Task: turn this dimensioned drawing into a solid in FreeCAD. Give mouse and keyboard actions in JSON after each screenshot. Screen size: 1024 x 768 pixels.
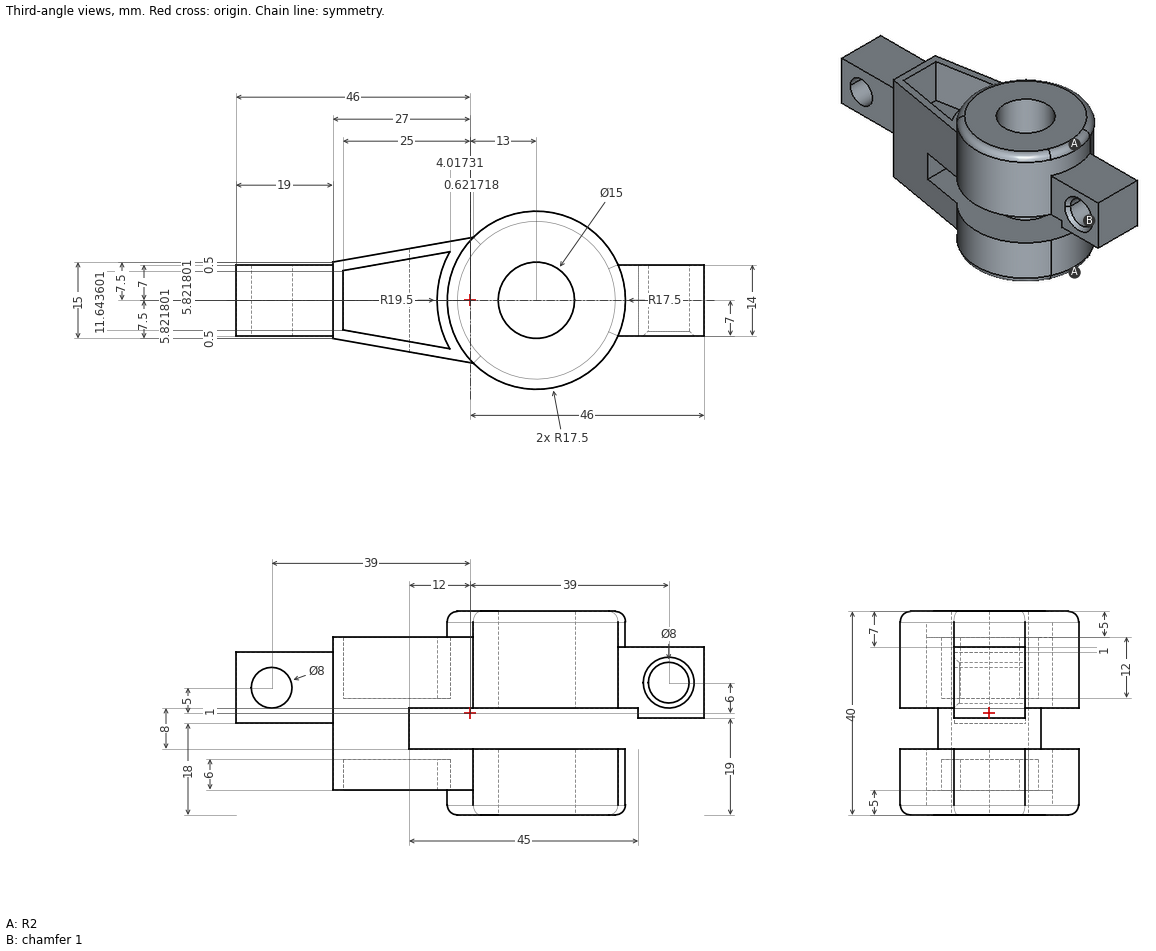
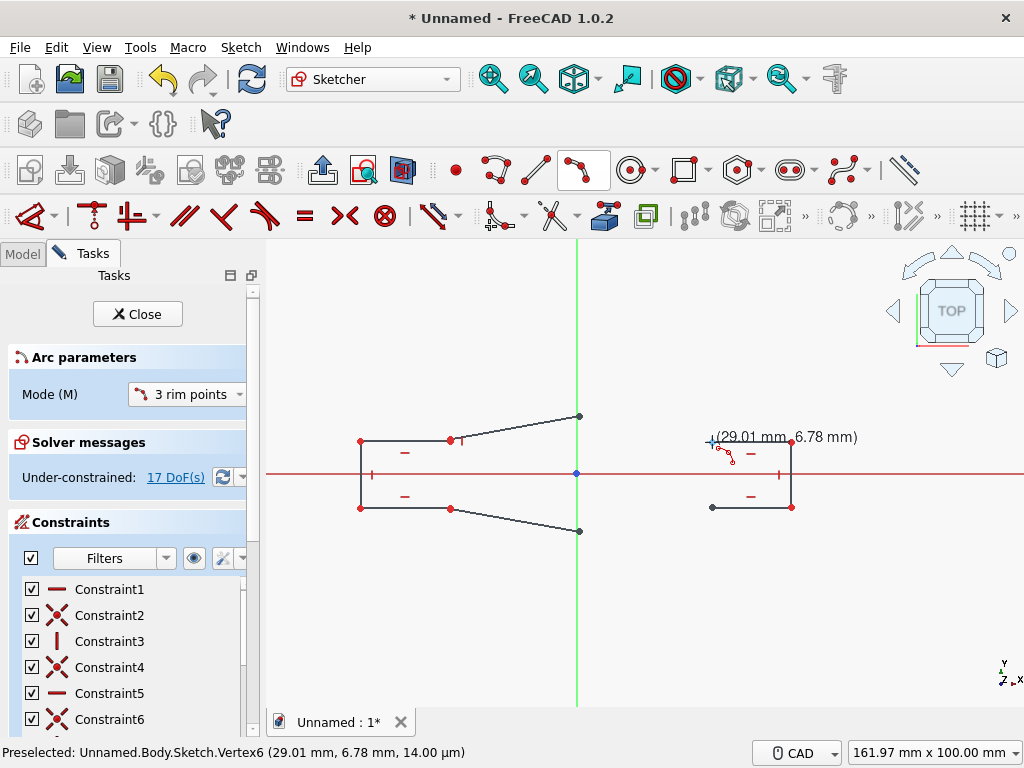
{"action": "scroll", "coordinate": [579, 416], "scroll_direction": "up", "scroll_amount": 9}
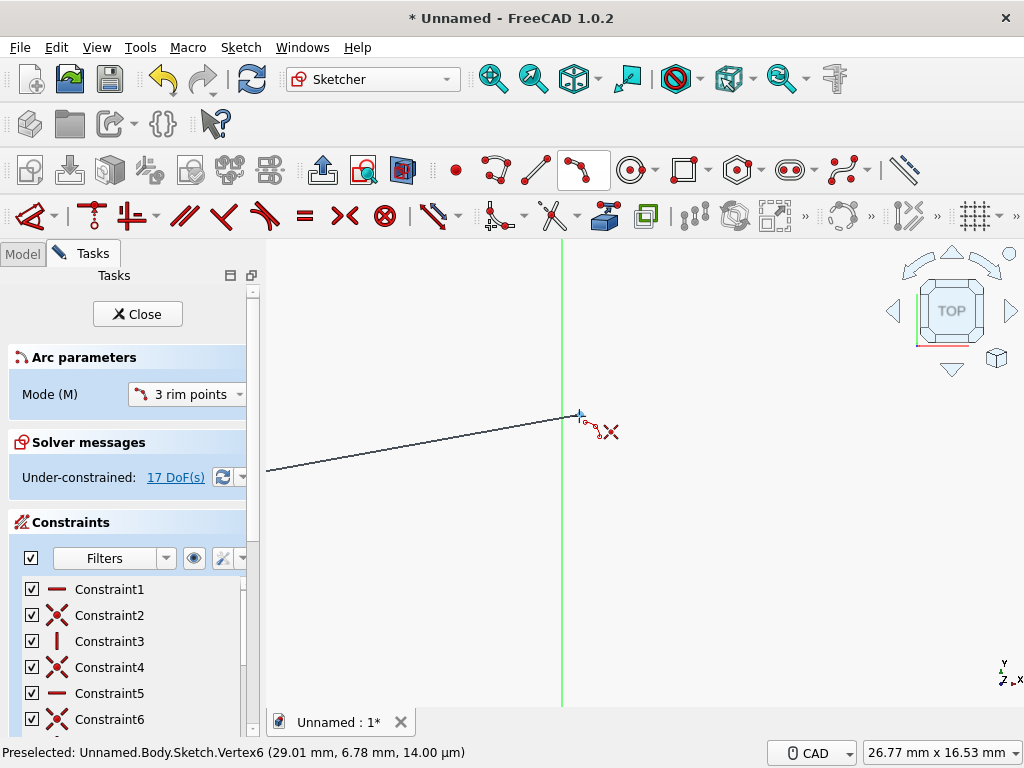
{"action": "left_click", "coordinate": [580, 415]}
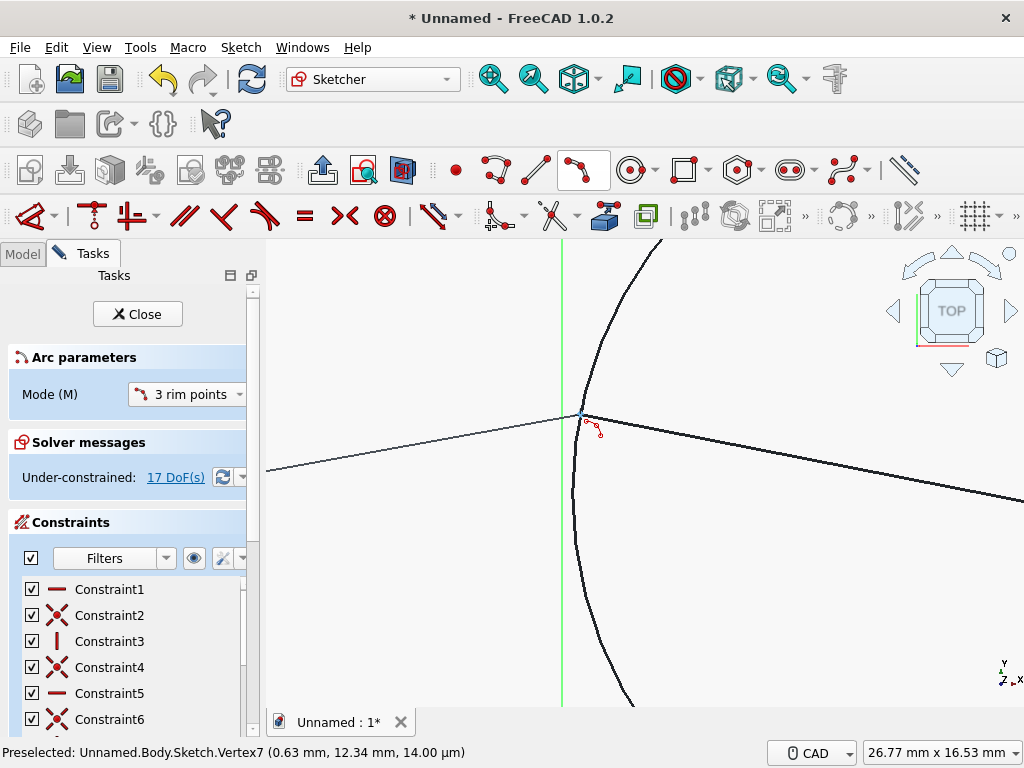
{"action": "scroll", "coordinate": [579, 415], "scroll_direction": "down", "scroll_amount": 9}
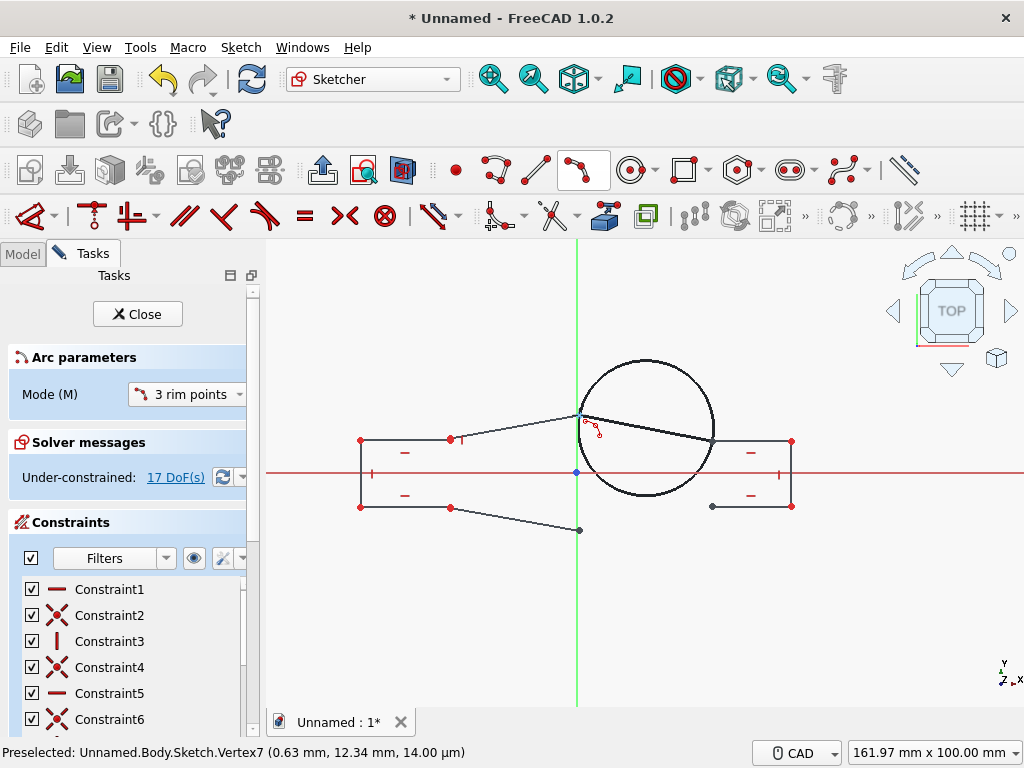
{"action": "left_click", "coordinate": [653, 393]}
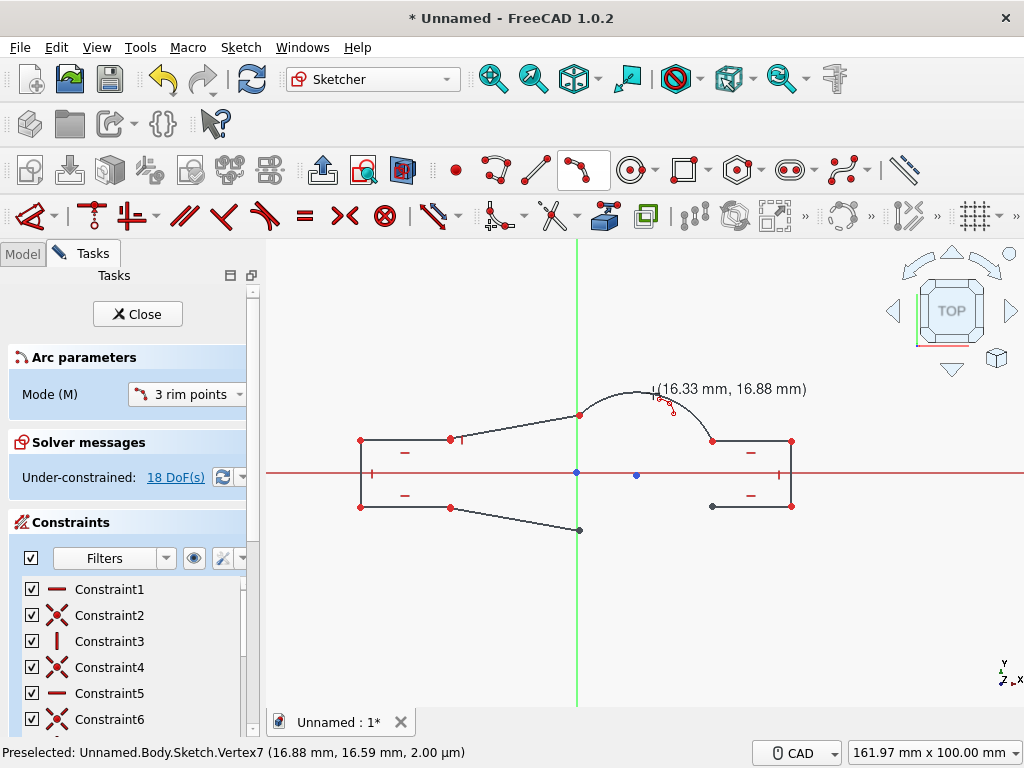
{"action": "scroll", "coordinate": [579, 531], "scroll_direction": "up", "scroll_amount": 9}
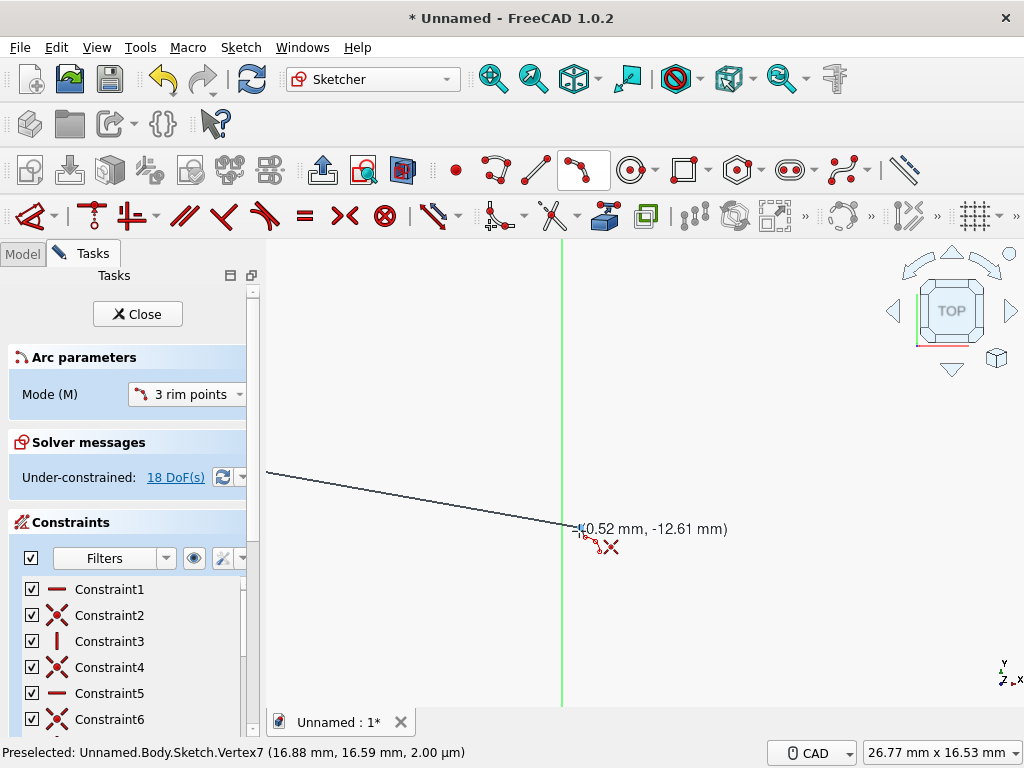
{"action": "left_click", "coordinate": [580, 528]}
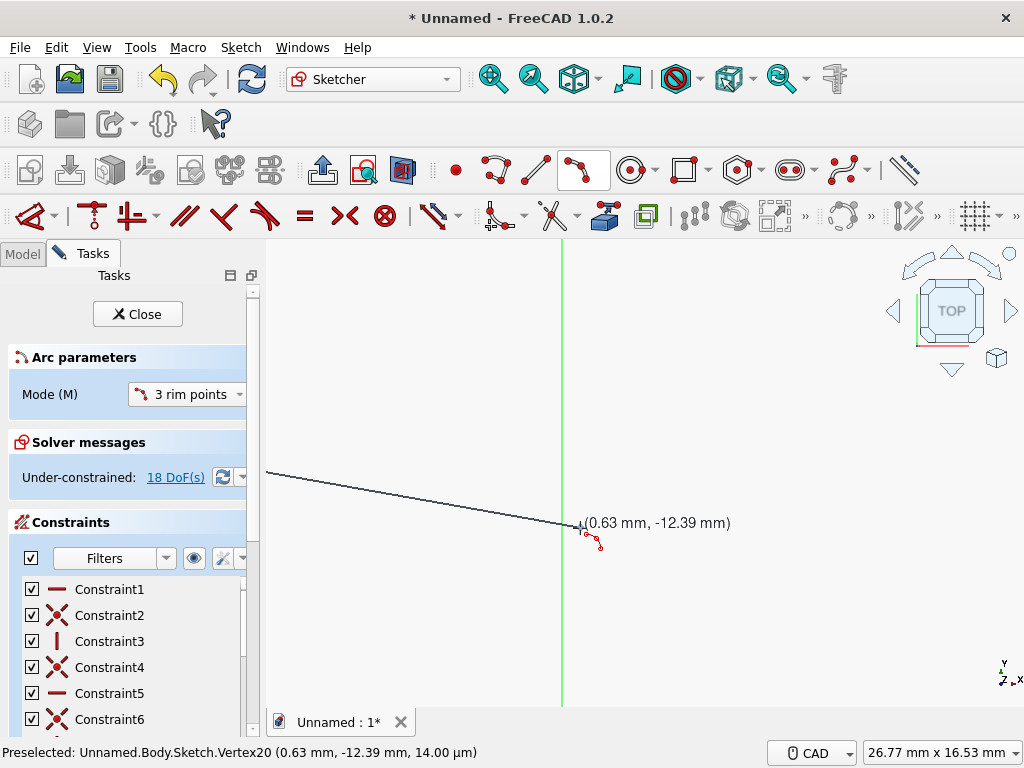
{"action": "scroll", "coordinate": [579, 532], "scroll_direction": "down", "scroll_amount": 9}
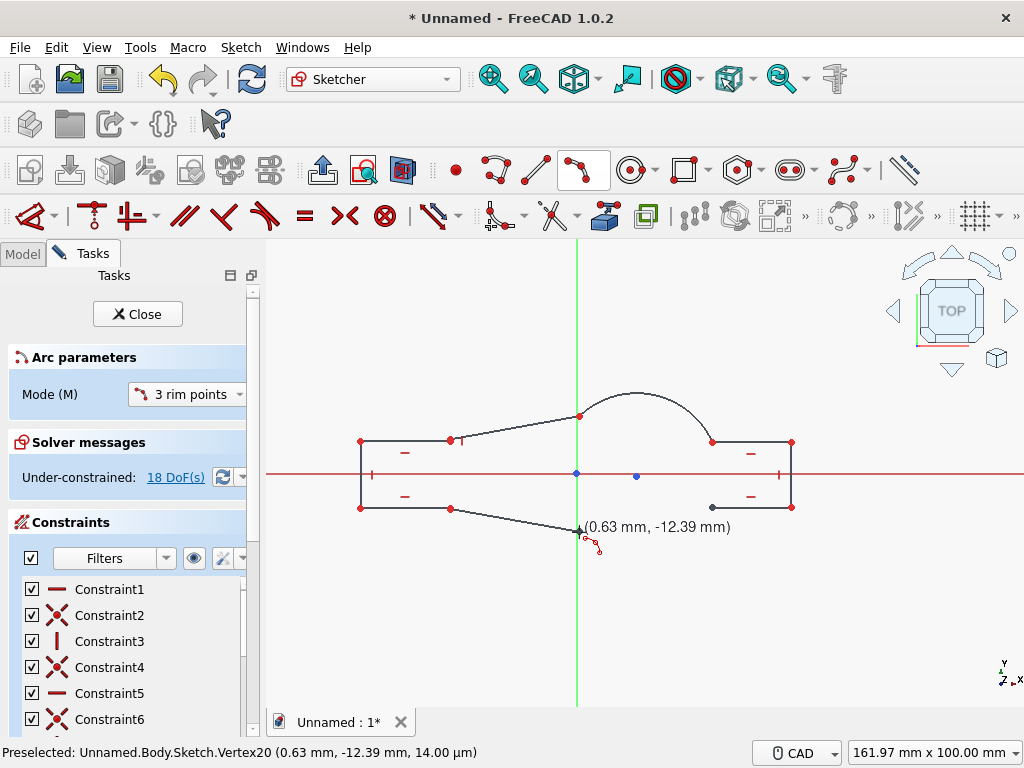
{"action": "left_click", "coordinate": [712, 508]}
{"action": "left_click", "coordinate": [653, 554]}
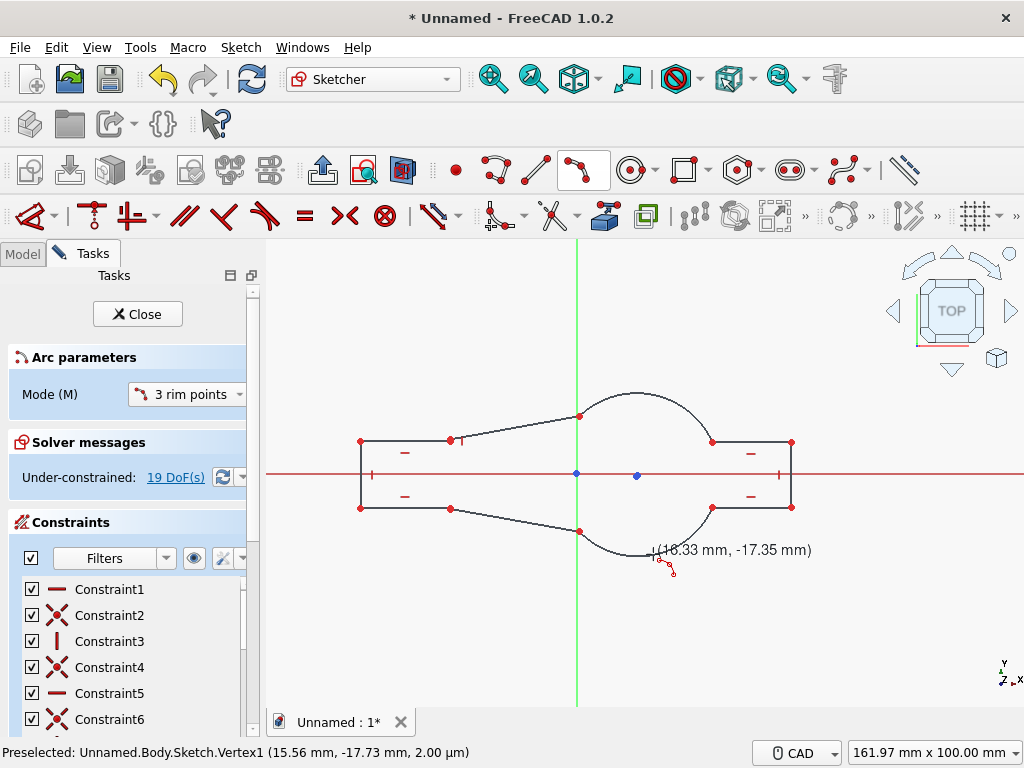
{"action": "left_click", "coordinate": [632, 170]}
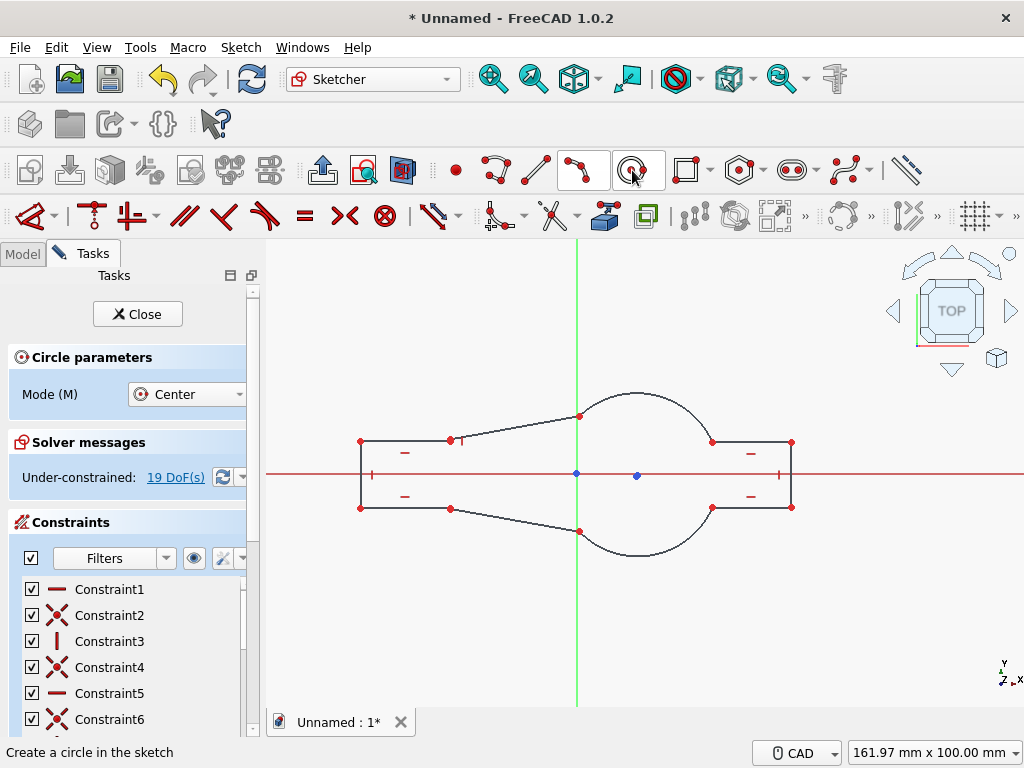
{"action": "left_click", "coordinate": [637, 474]}
{"action": "left_click", "coordinate": [662, 449]}
{"action": "key", "text": "Escape"}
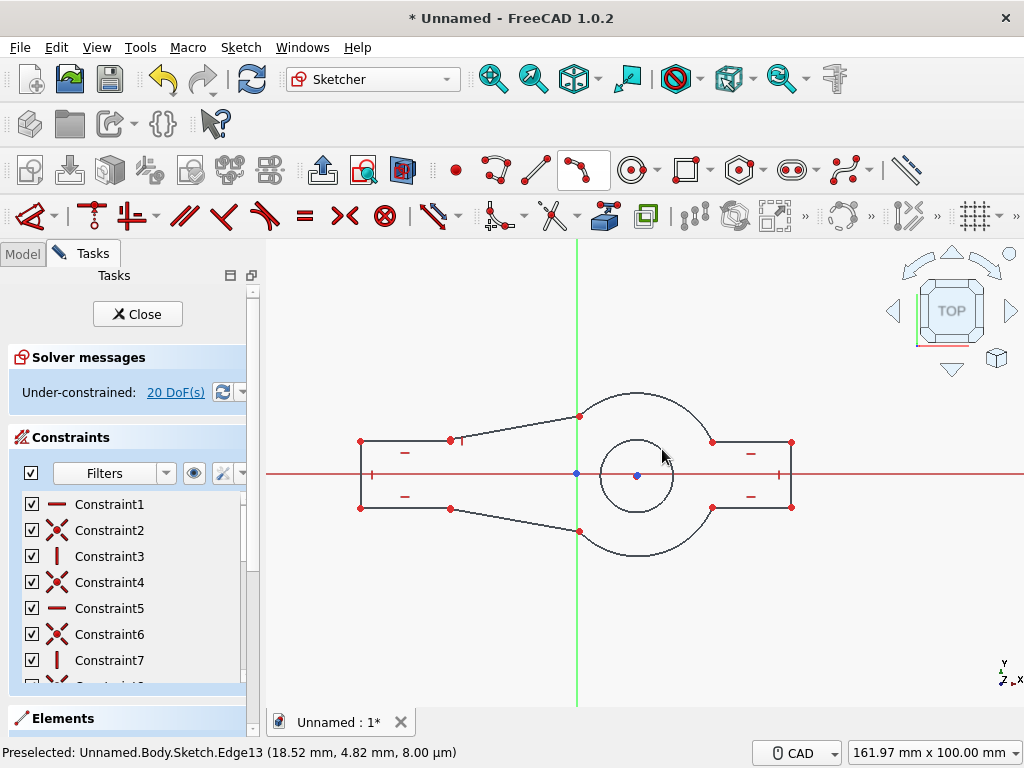
{"action": "scroll", "coordinate": [451, 509], "scroll_direction": "up", "scroll_amount": 13}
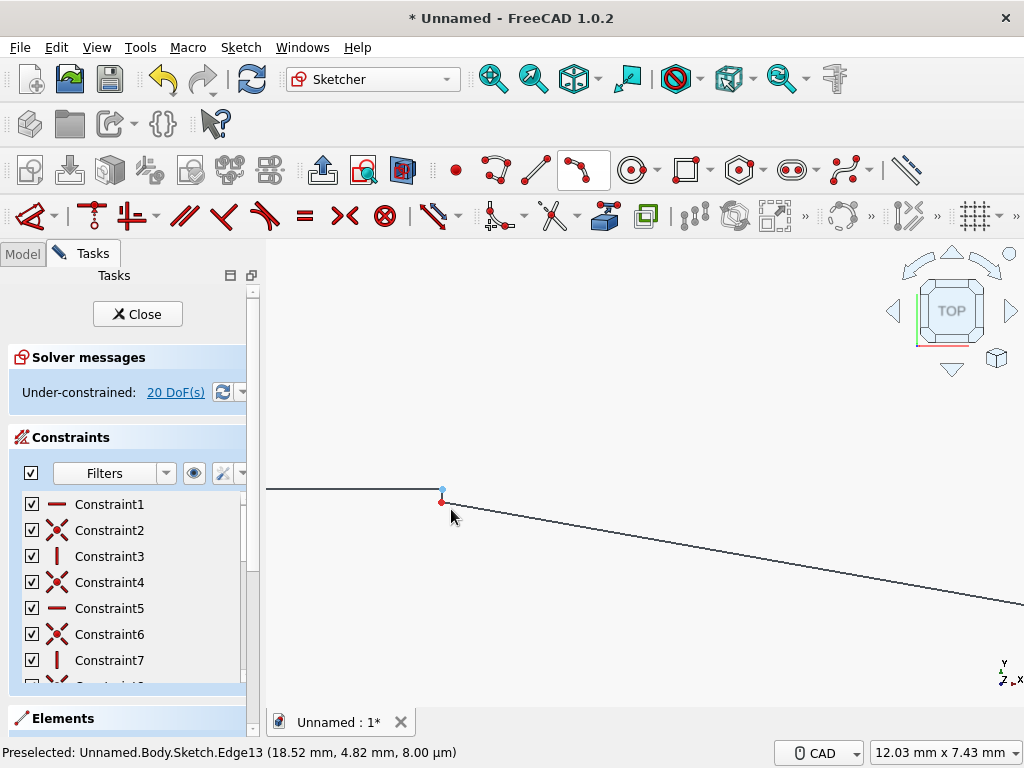
{"action": "left_click", "coordinate": [442, 496]}